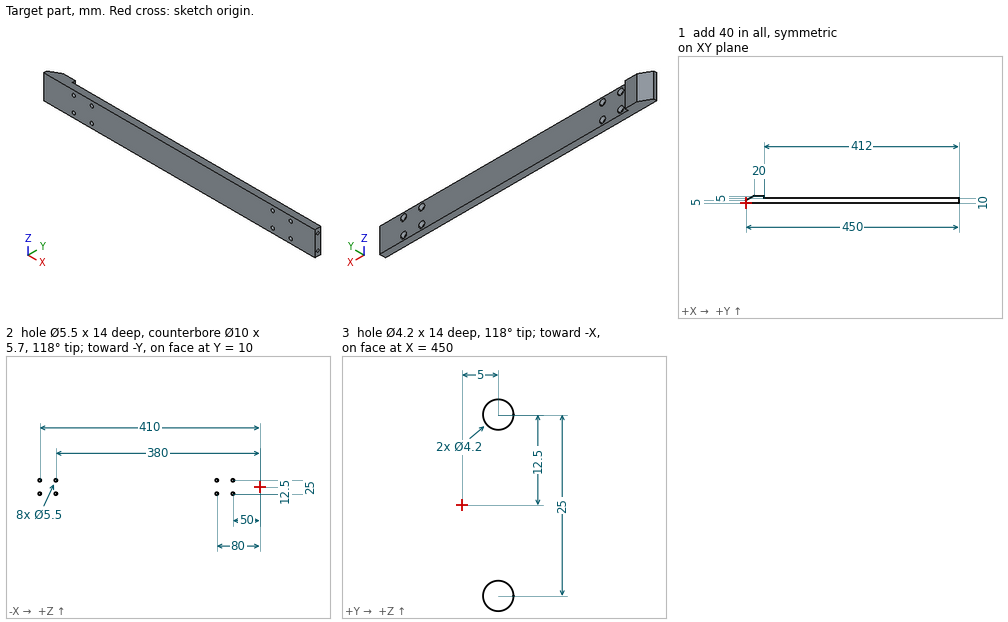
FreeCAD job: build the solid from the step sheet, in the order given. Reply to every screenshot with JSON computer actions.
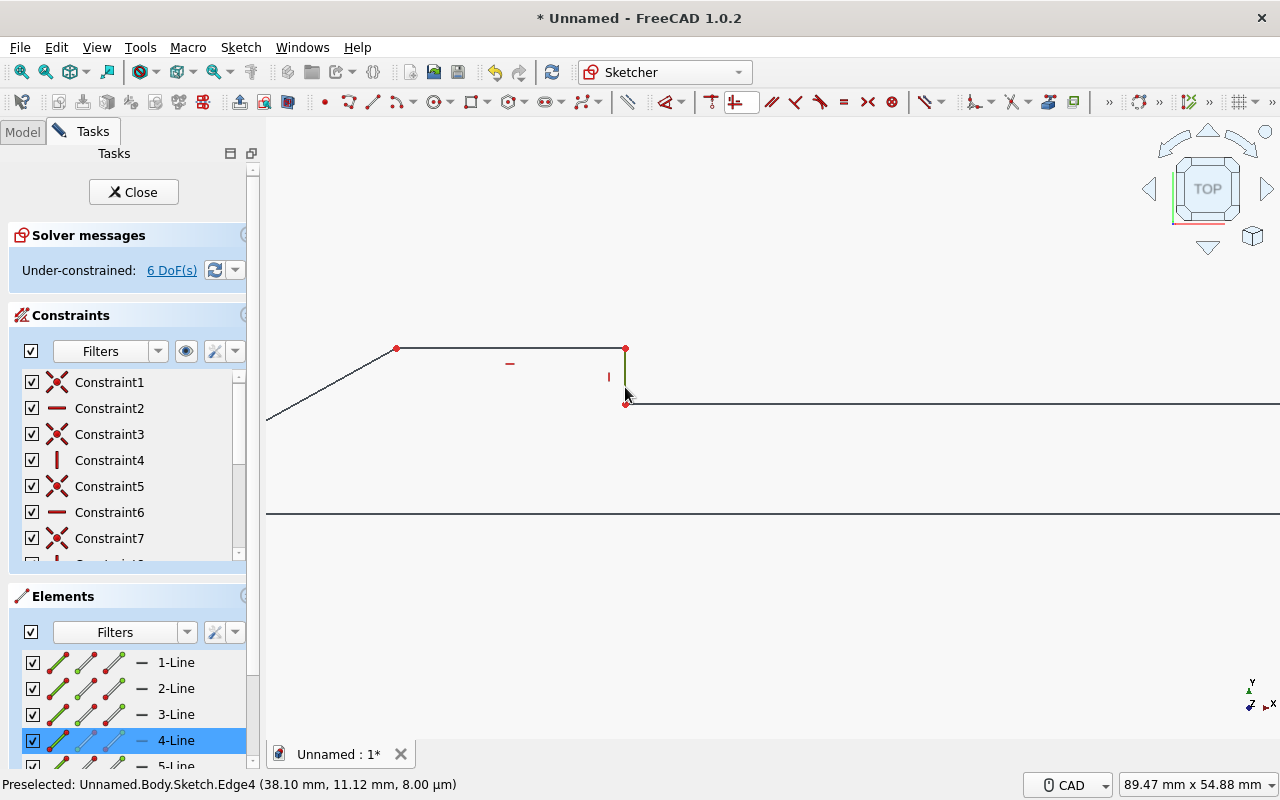
{"action": "key", "text": "i"}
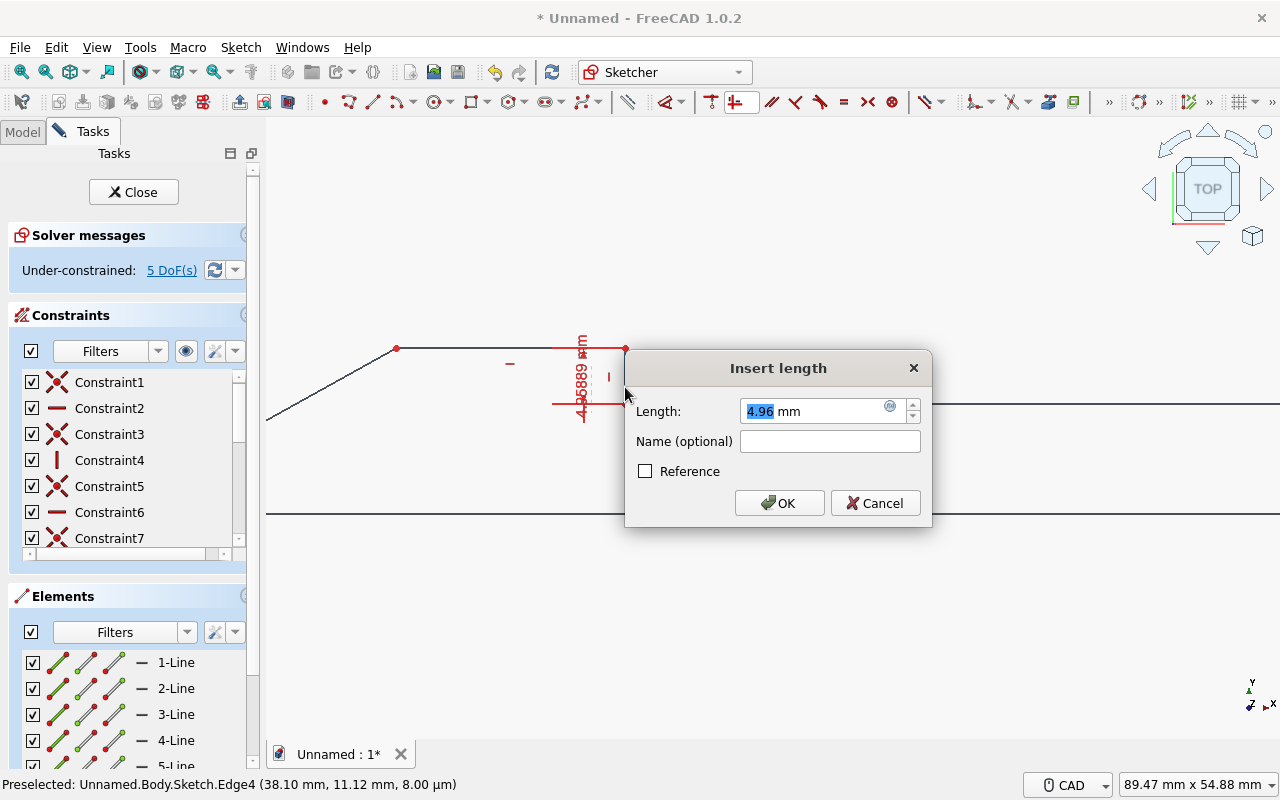
{"action": "type", "text": "5"}
{"action": "key", "text": "Return"}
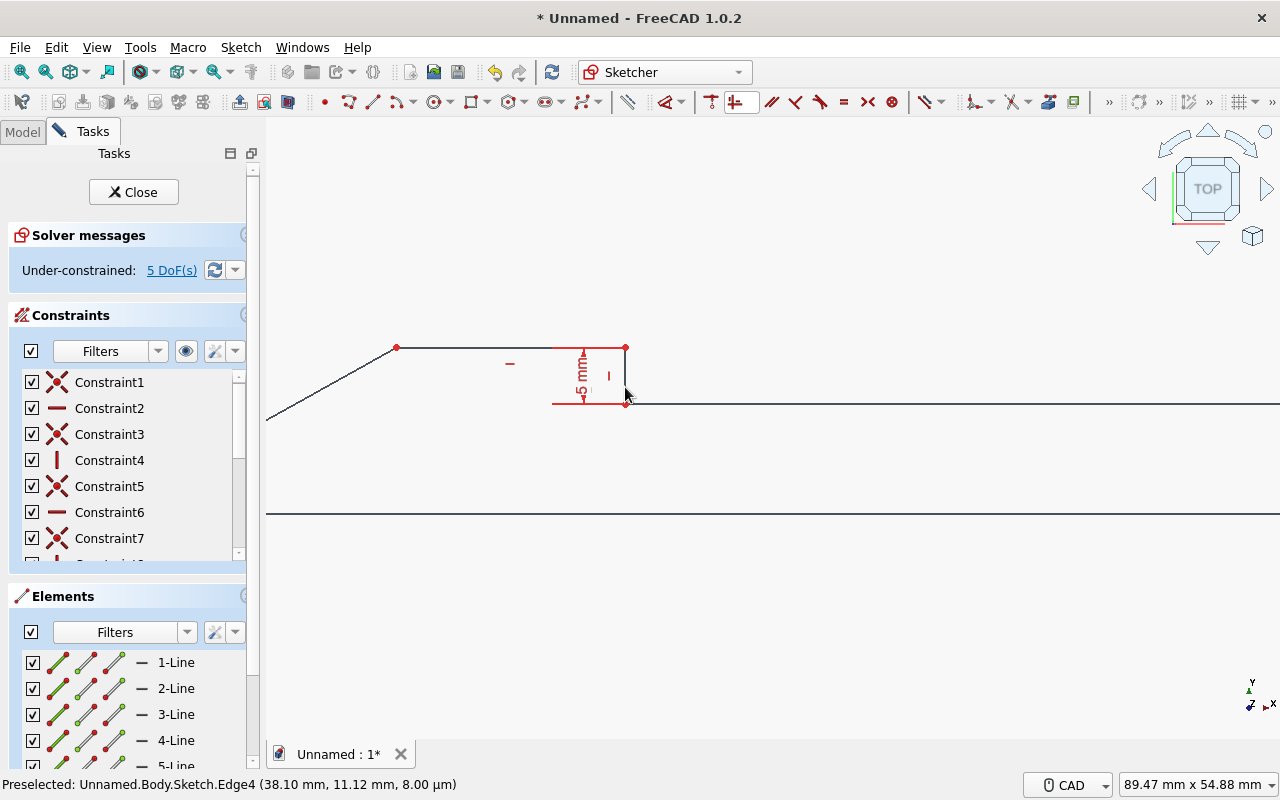
{"action": "scroll", "coordinate": [450, 428], "scroll_direction": "down", "scroll_amount": 11}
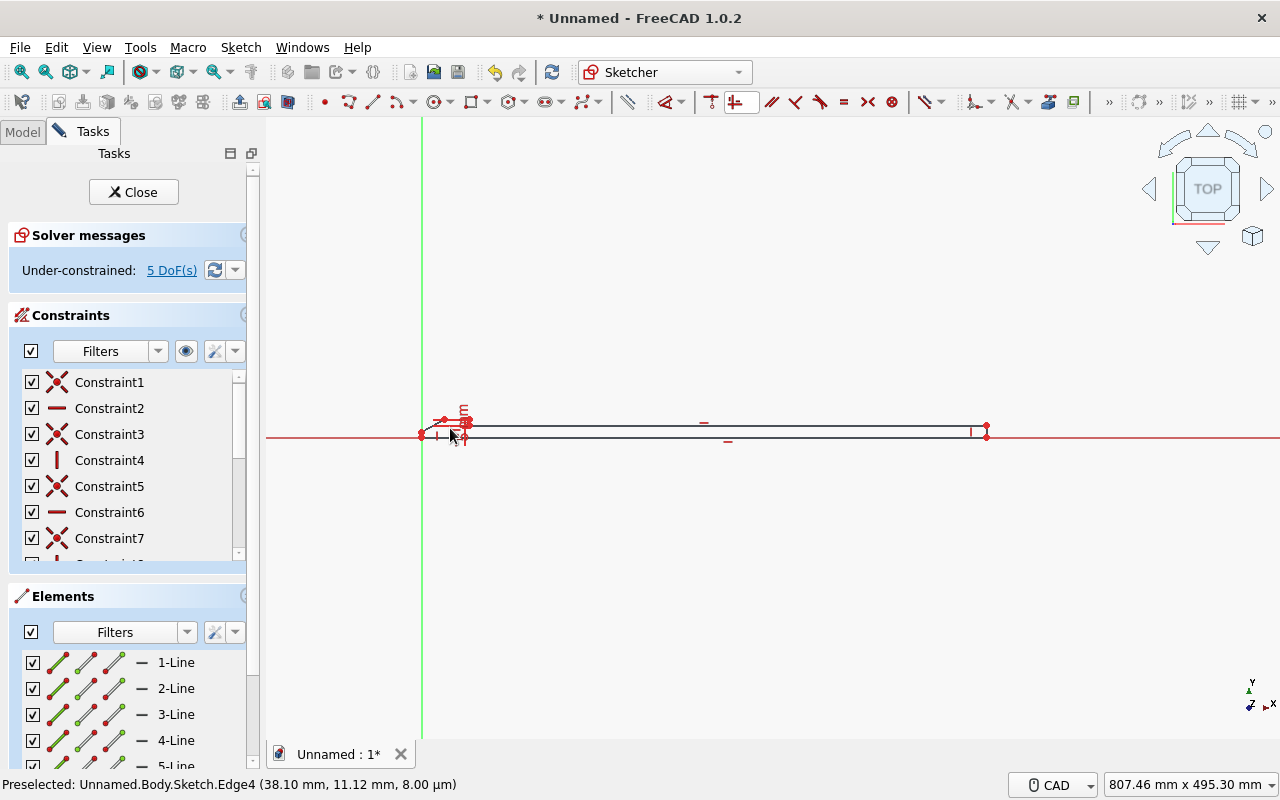
{"action": "scroll", "coordinate": [422, 434], "scroll_direction": "up", "scroll_amount": 11}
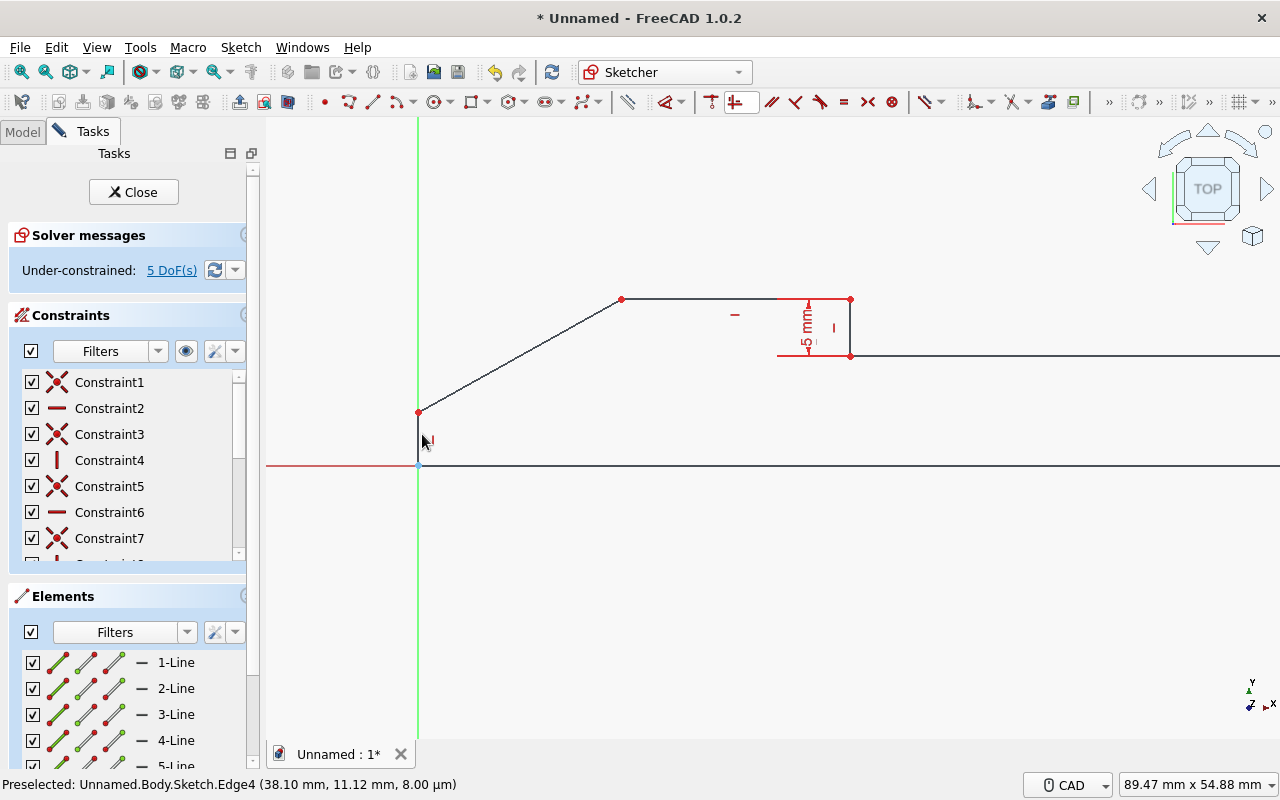
{"action": "left_click", "coordinate": [418, 429]}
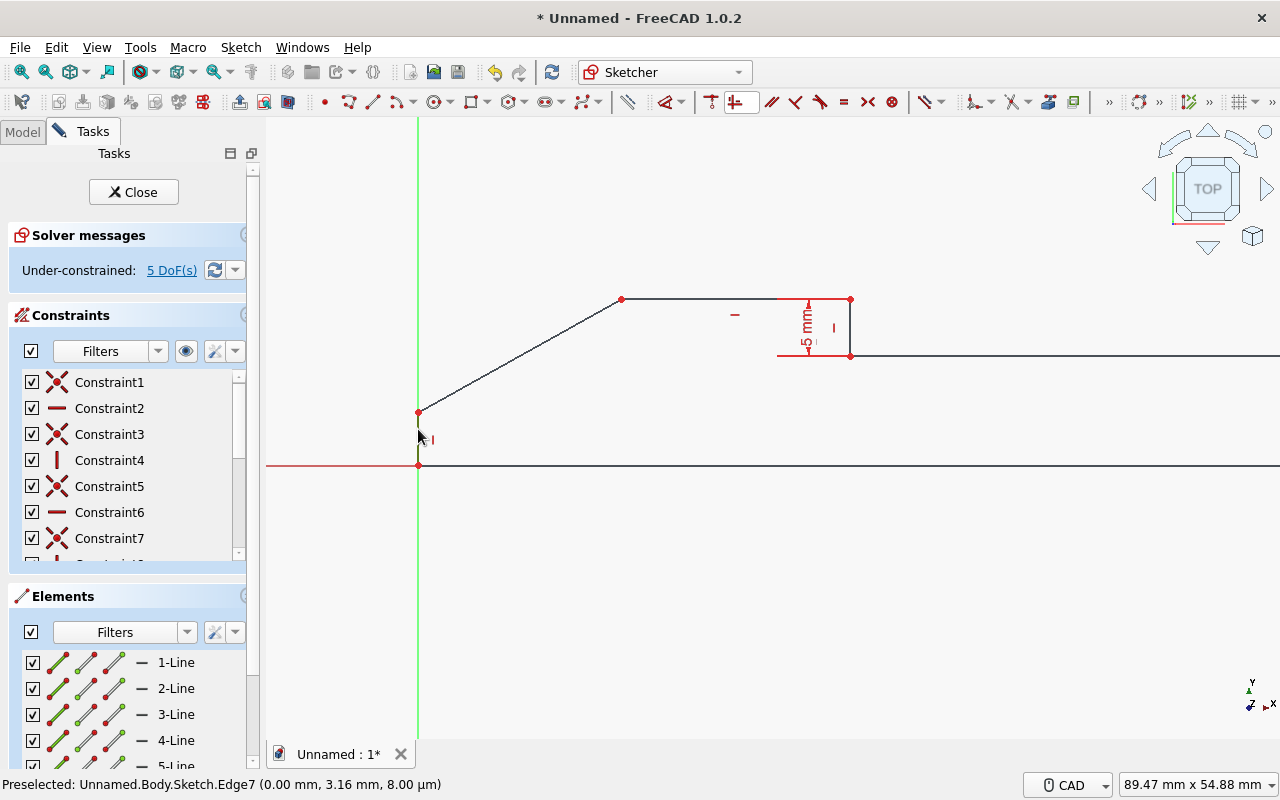
{"action": "key", "text": "i"}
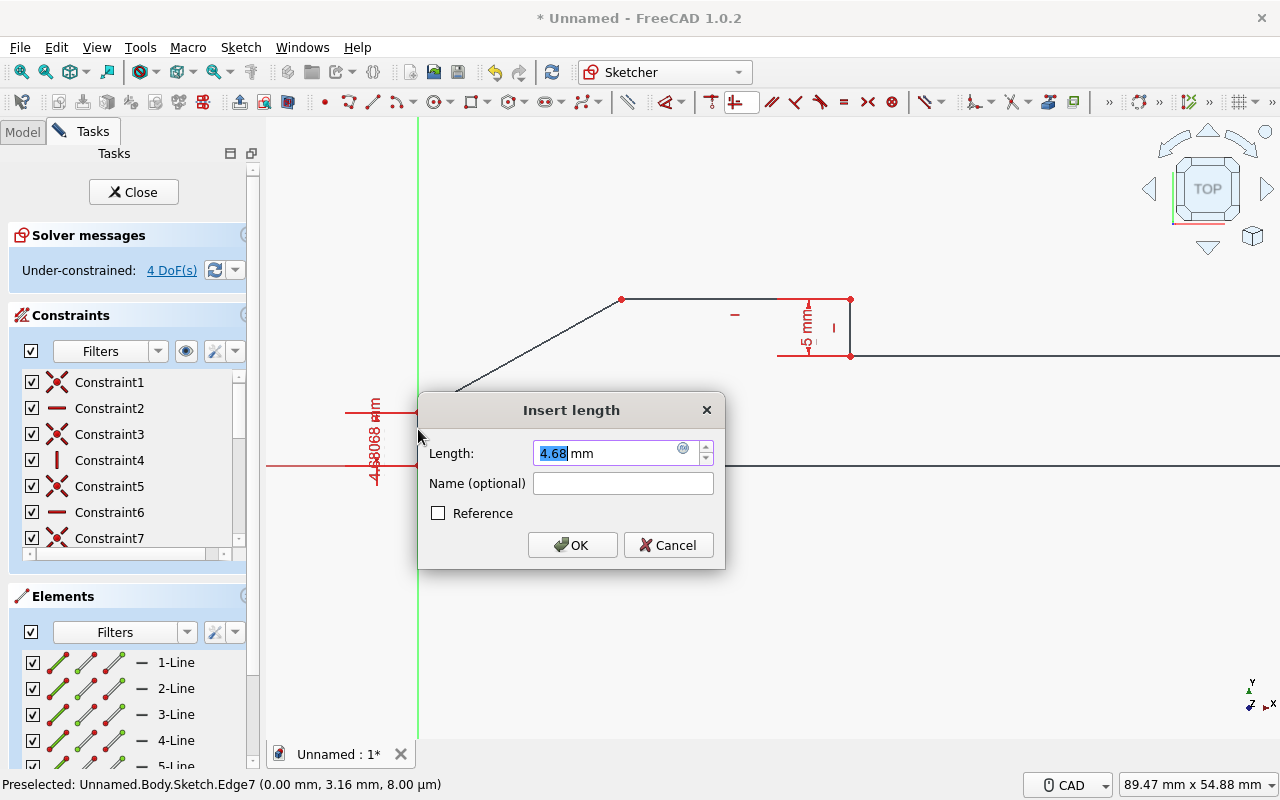
{"action": "type", "text": "5"}
{"action": "key", "text": "Return"}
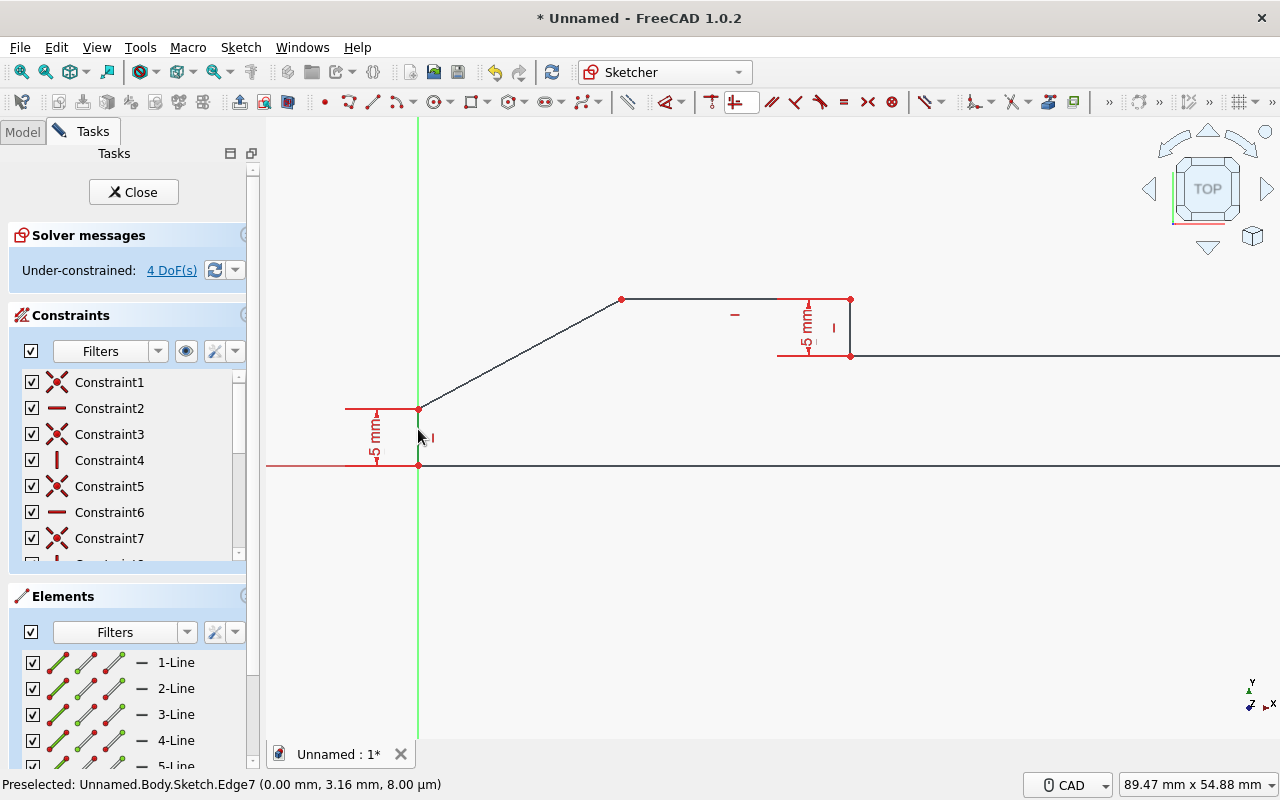
{"action": "scroll", "coordinate": [422, 434], "scroll_direction": "down", "scroll_amount": 11}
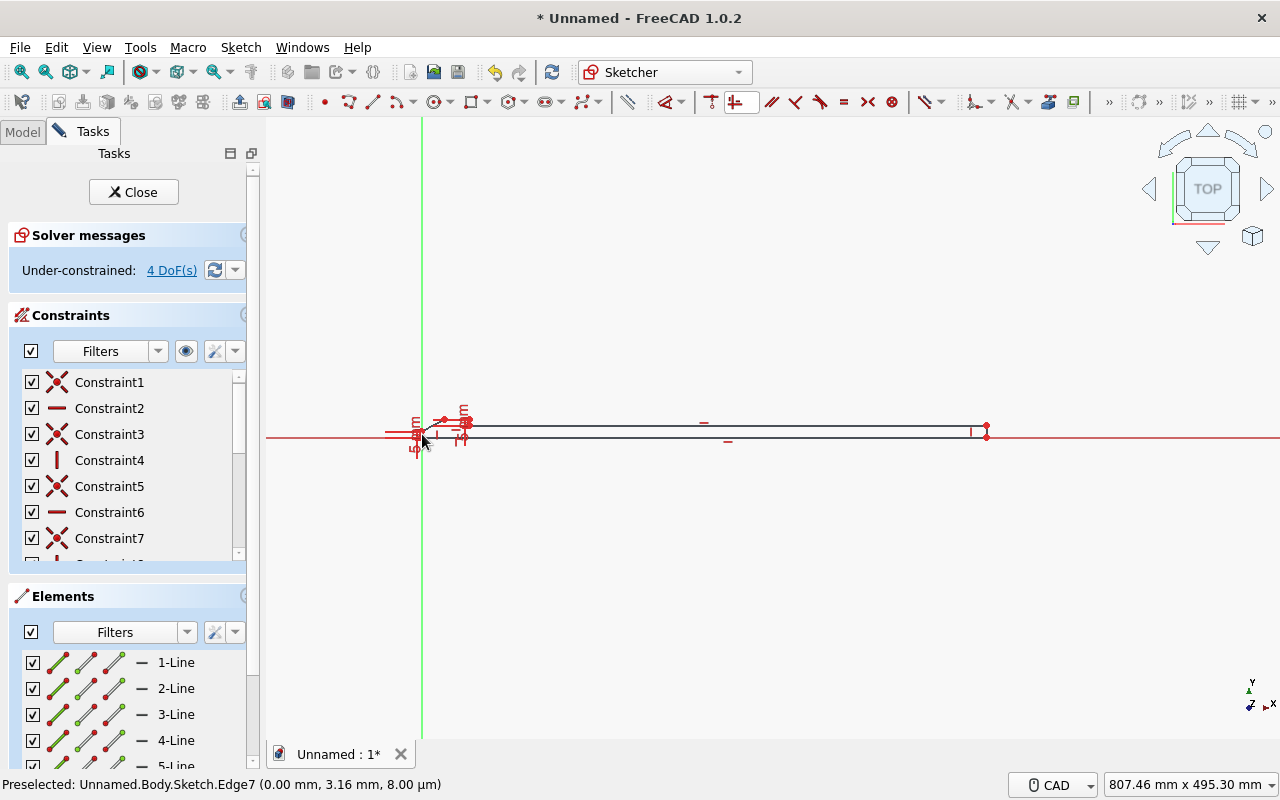
{"action": "scroll", "coordinate": [987, 434], "scroll_direction": "up", "scroll_amount": 7}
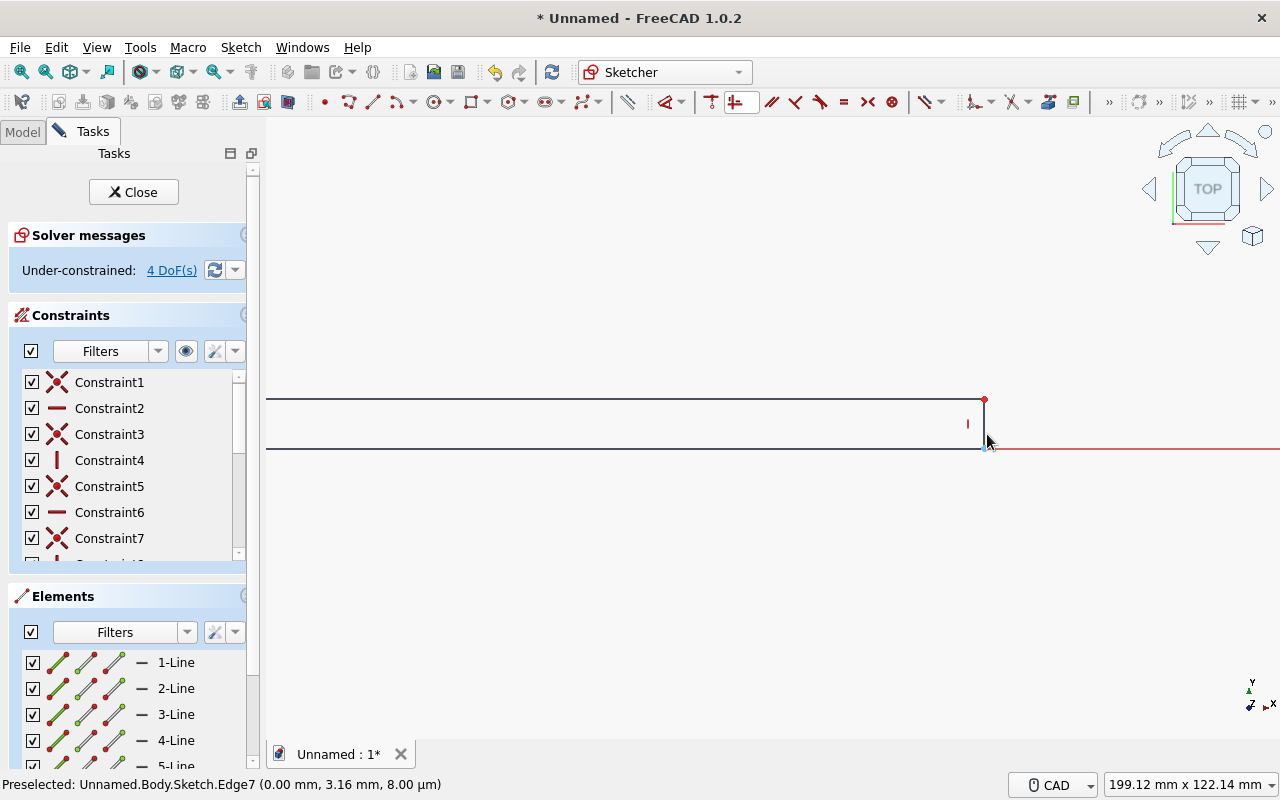
{"action": "left_click", "coordinate": [984, 434]}